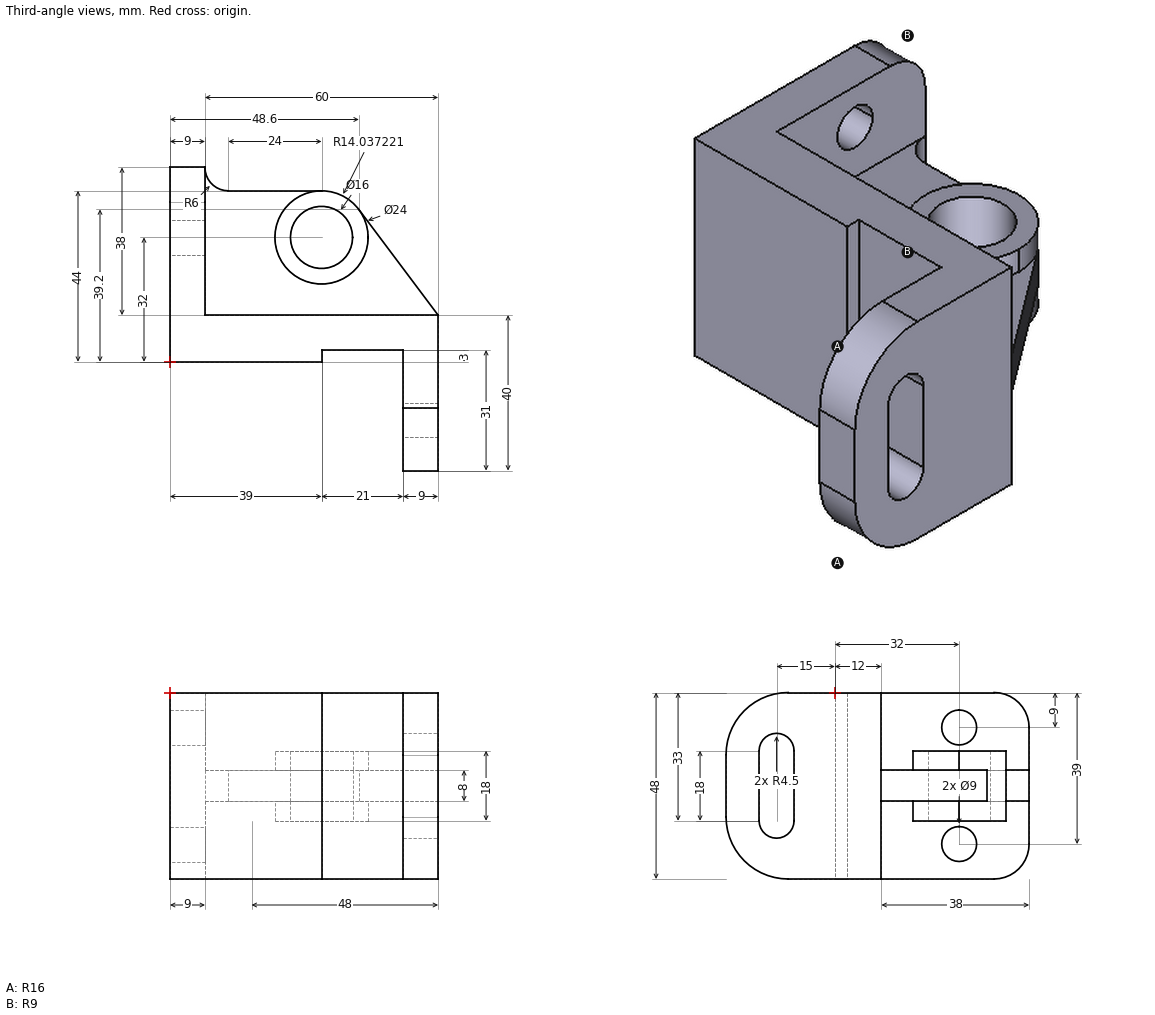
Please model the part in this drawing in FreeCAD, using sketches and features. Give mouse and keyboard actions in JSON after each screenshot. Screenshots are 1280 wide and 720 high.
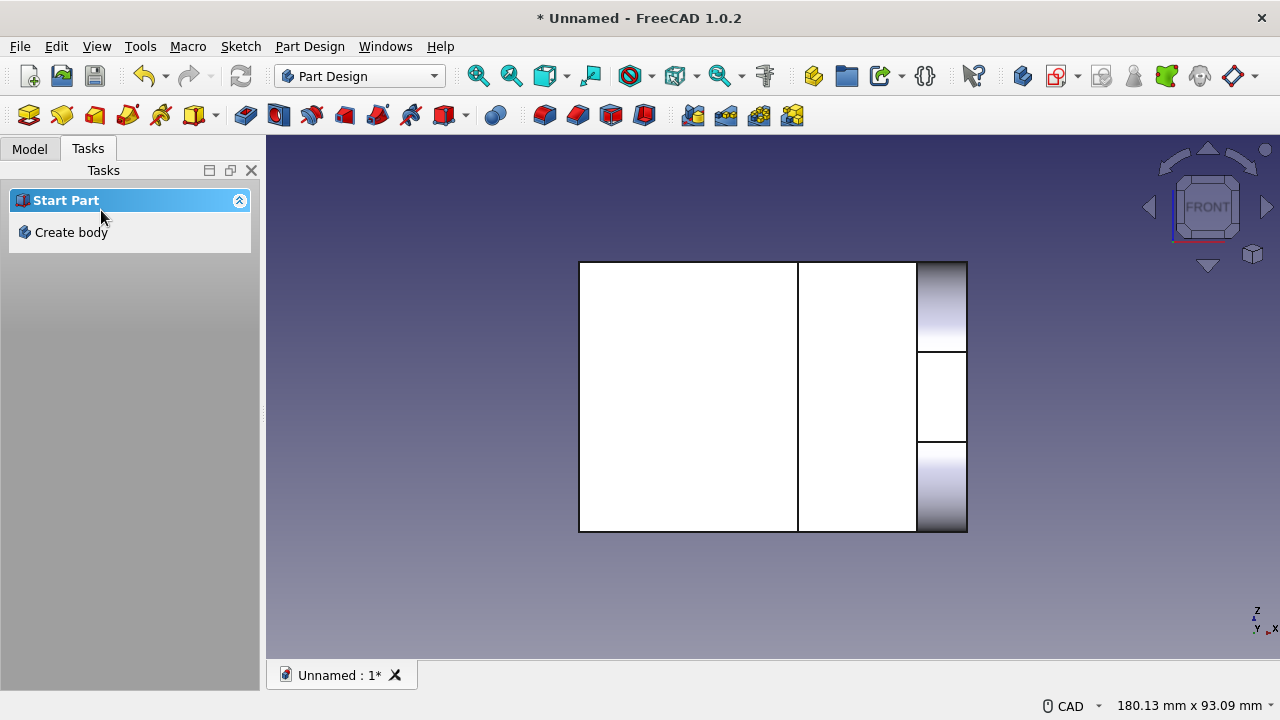
{"action": "key", "text": "0"}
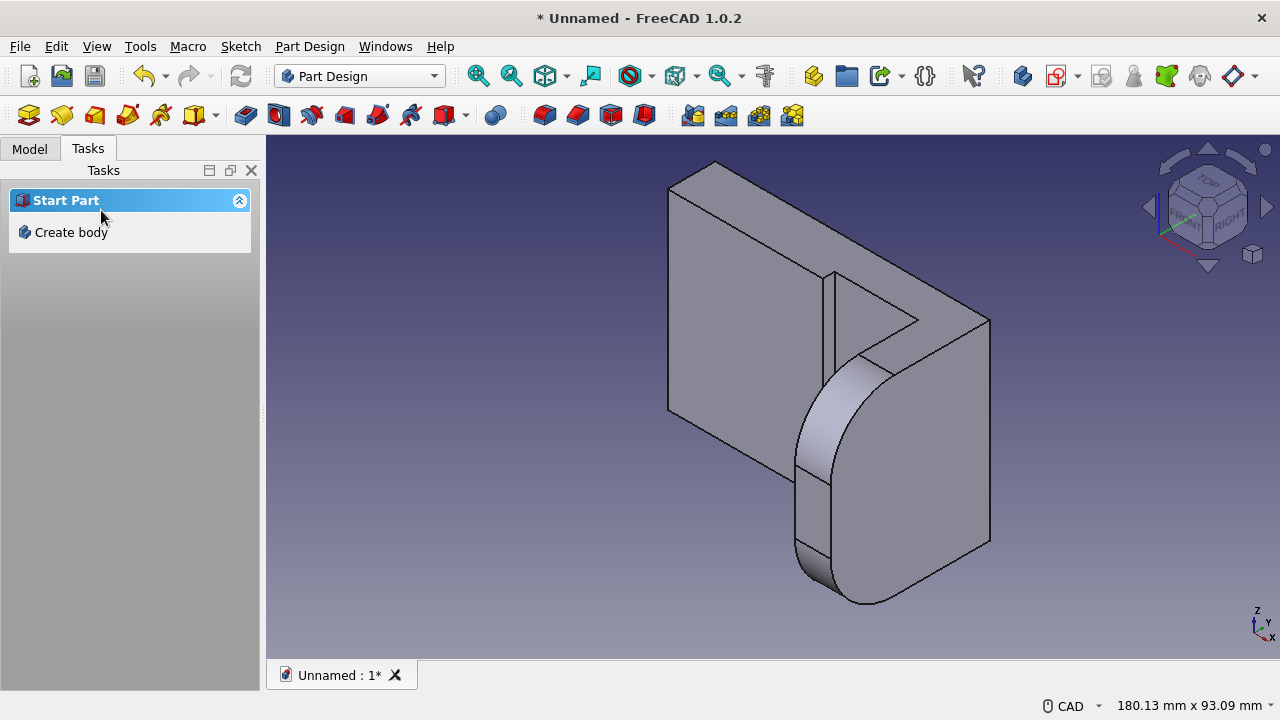
{"action": "left_click", "coordinate": [910, 475]}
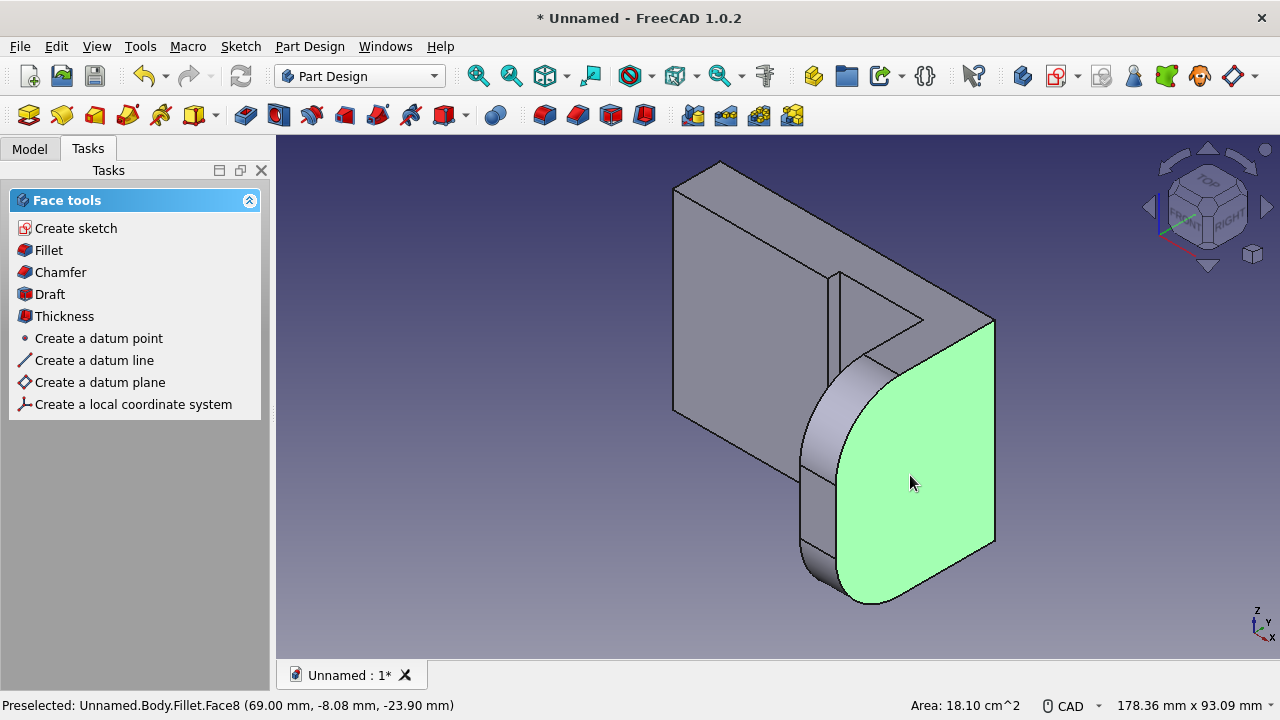
{"action": "left_click", "coordinate": [1056, 76]}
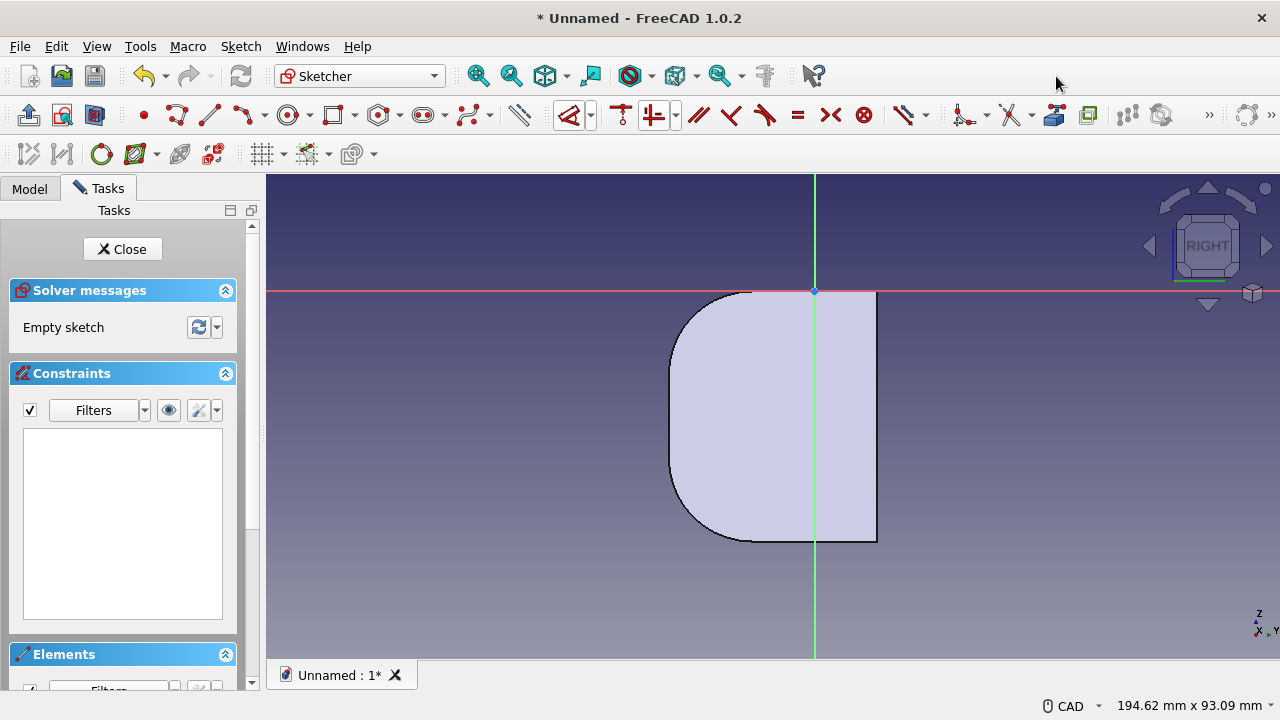
{"action": "scroll", "coordinate": [885, 334], "scroll_direction": "up", "scroll_amount": 2}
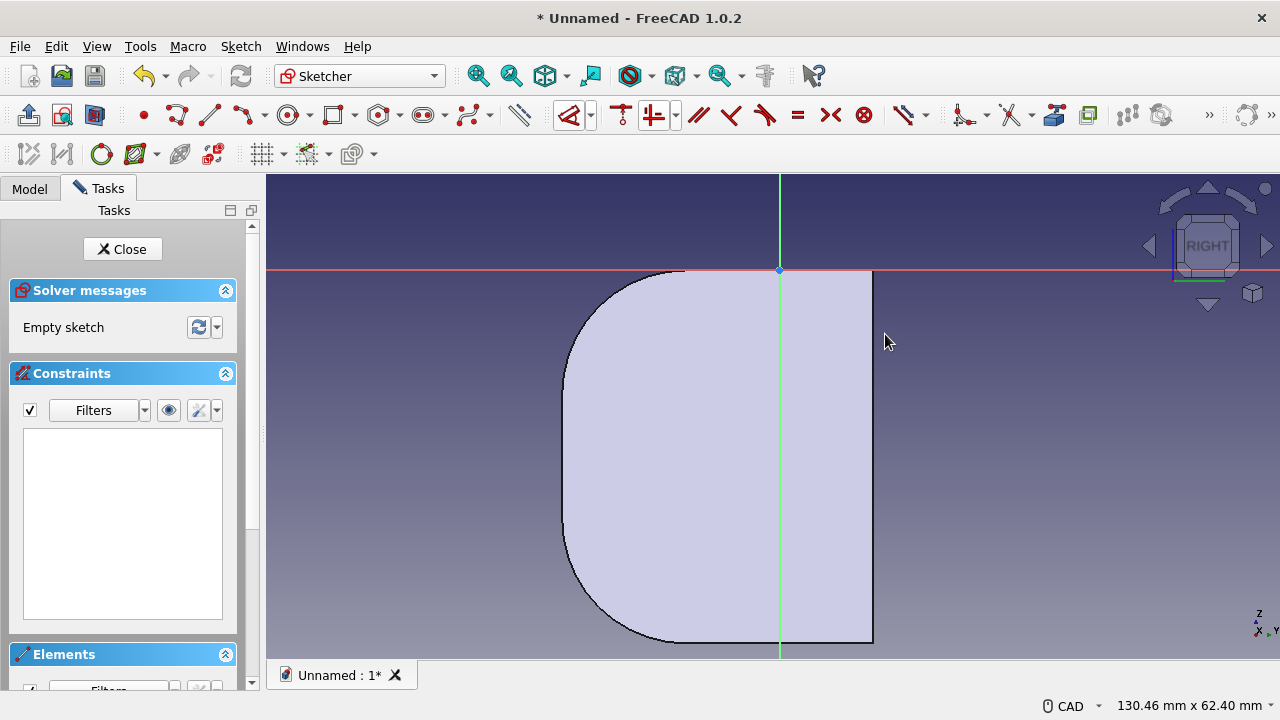
{"action": "key", "text": "g s"}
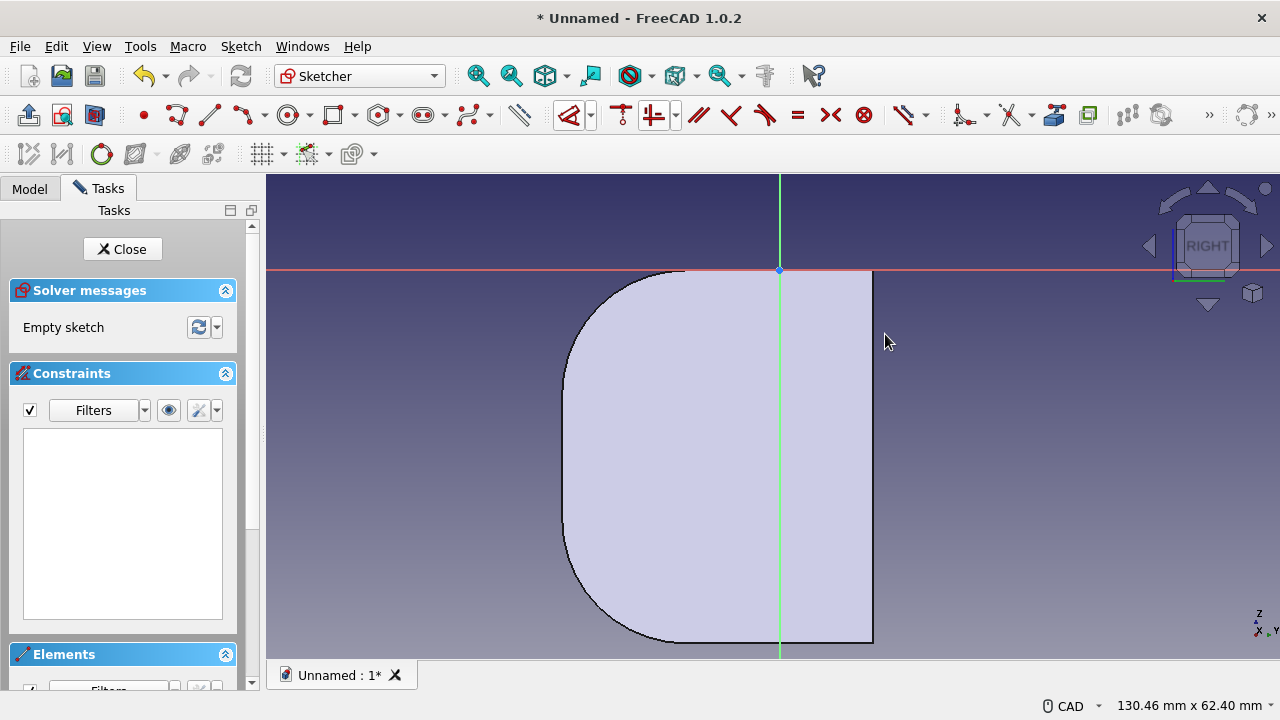
{"action": "left_click", "coordinate": [663, 527]}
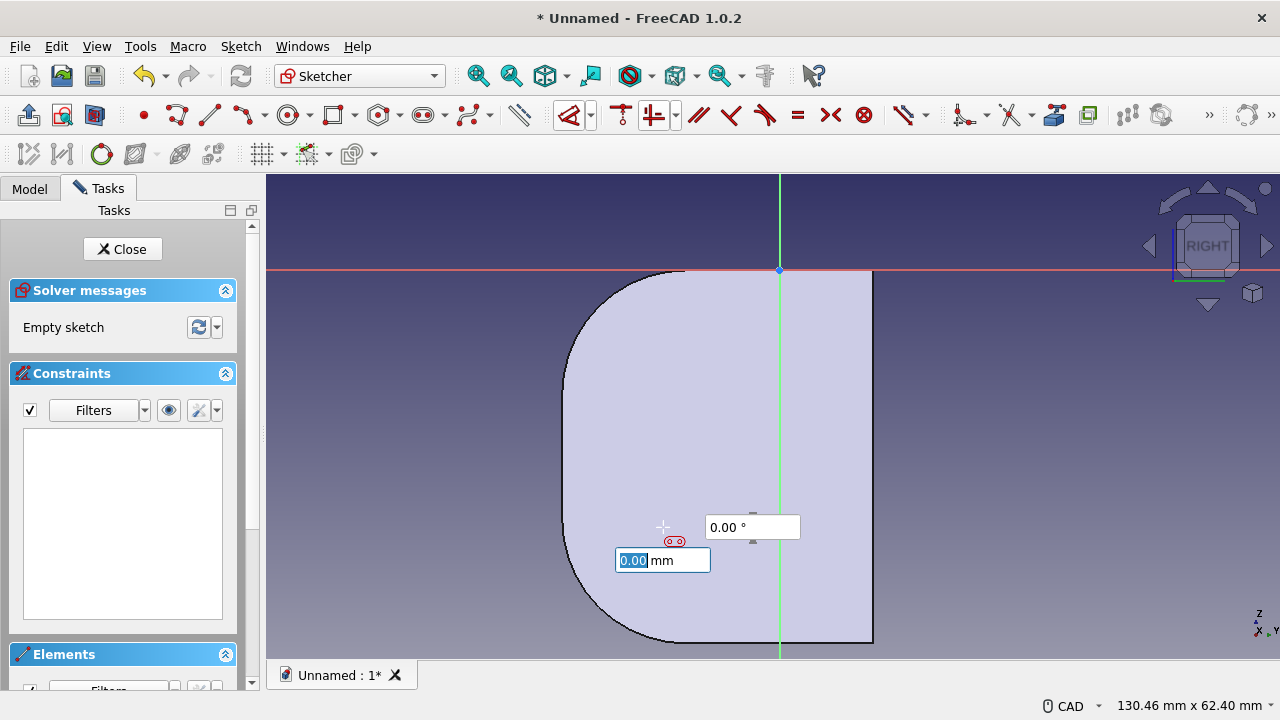
{"action": "left_click", "coordinate": [663, 387]}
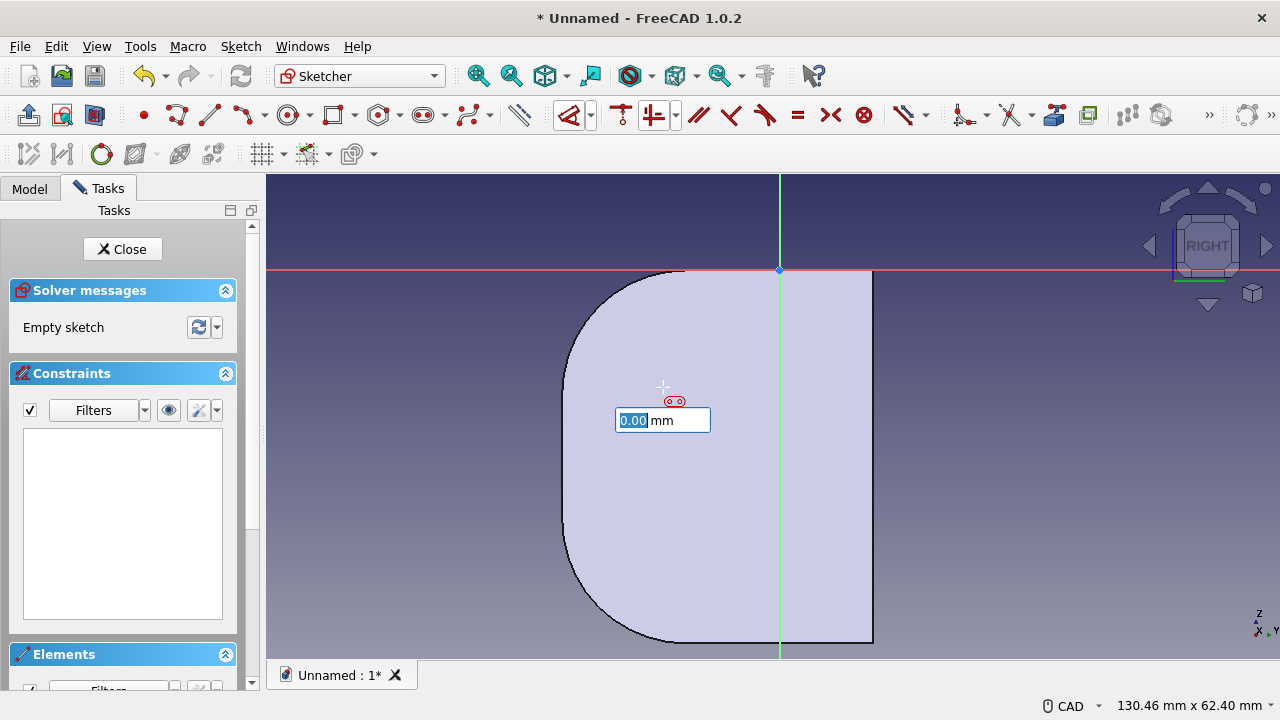
{"action": "left_click", "coordinate": [698, 457]}
{"action": "key", "text": "Escape"}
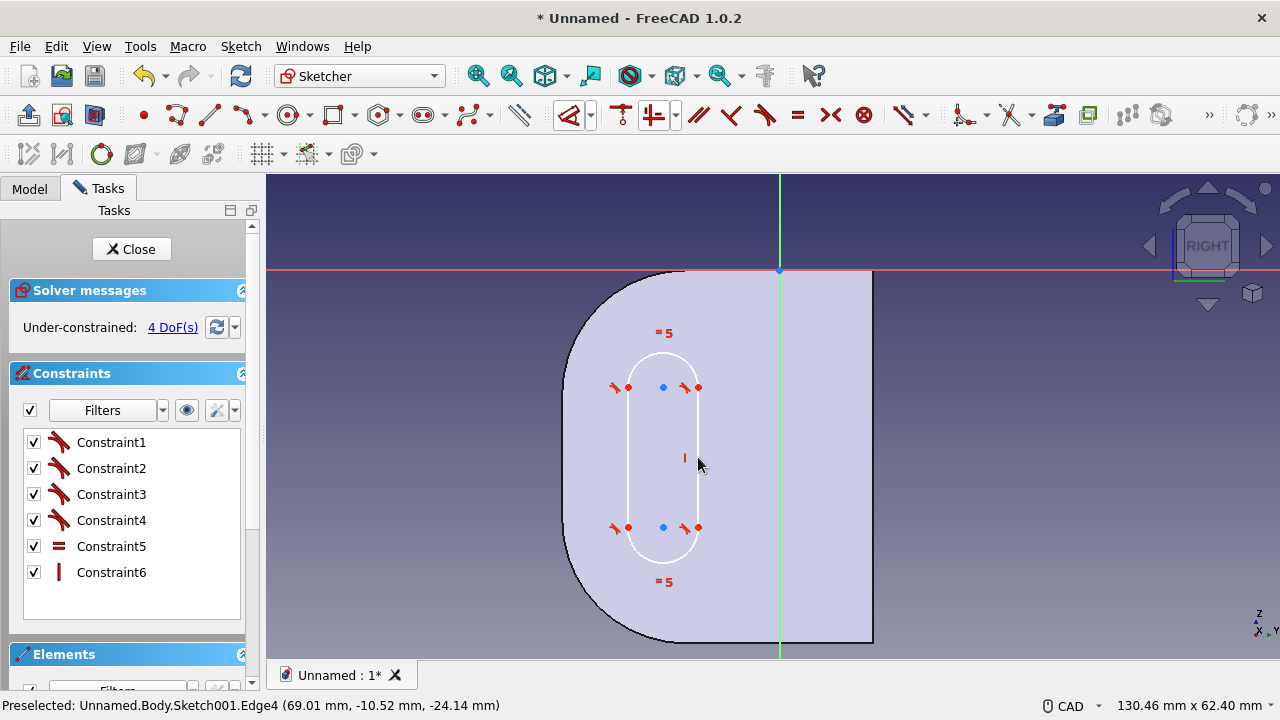
{"action": "left_click", "coordinate": [568, 116]}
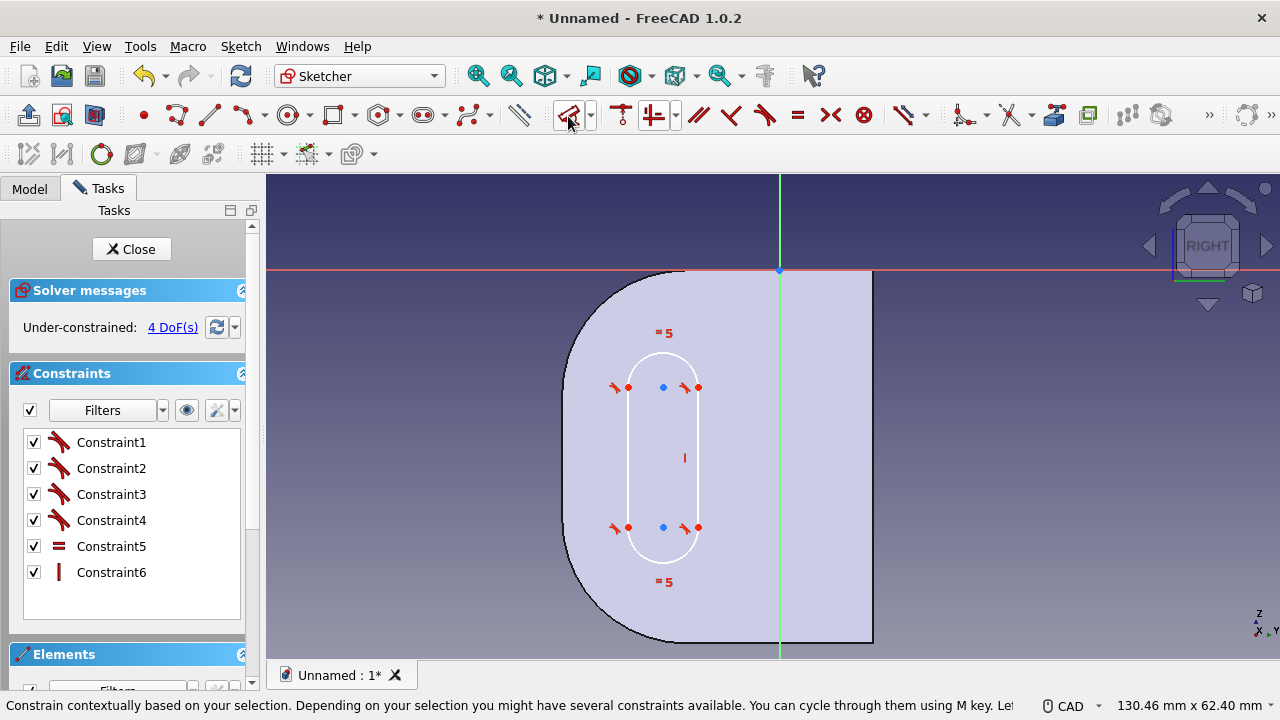
{"action": "left_click", "coordinate": [642, 556]}
{"action": "left_click", "coordinate": [623, 582]}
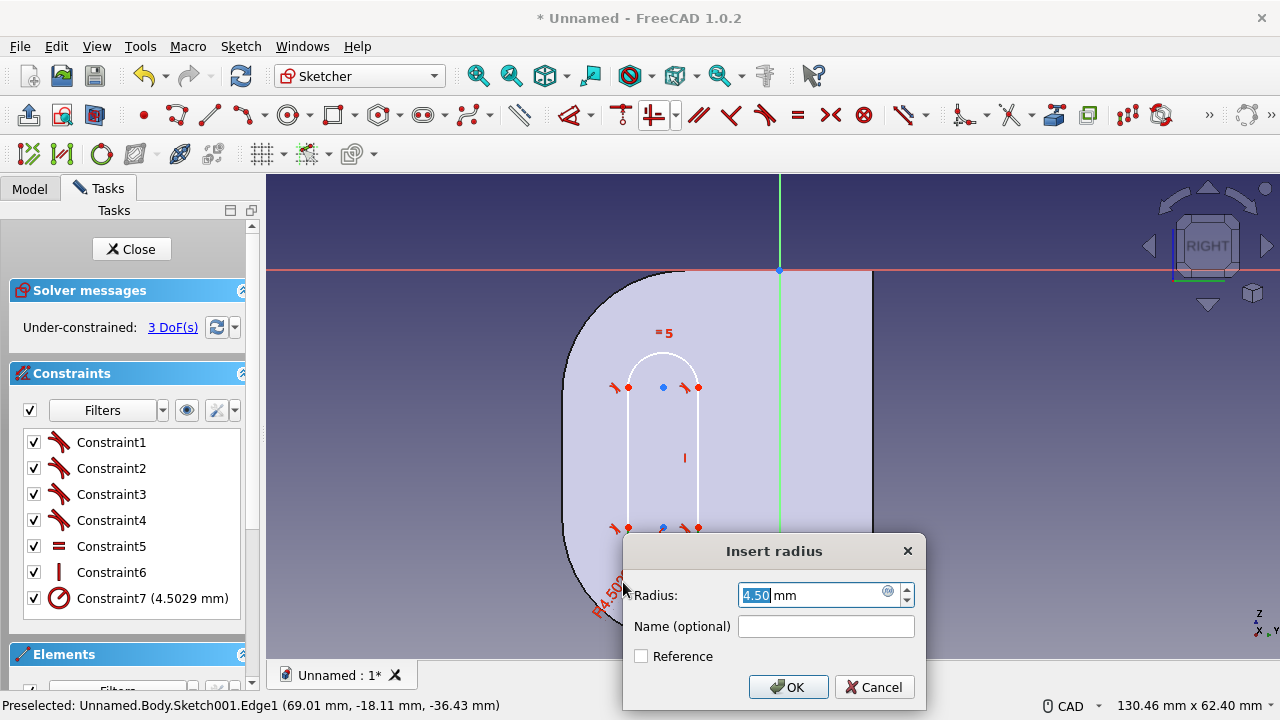
{"action": "type", "text": "4.5"}
{"action": "key", "text": "Return"}